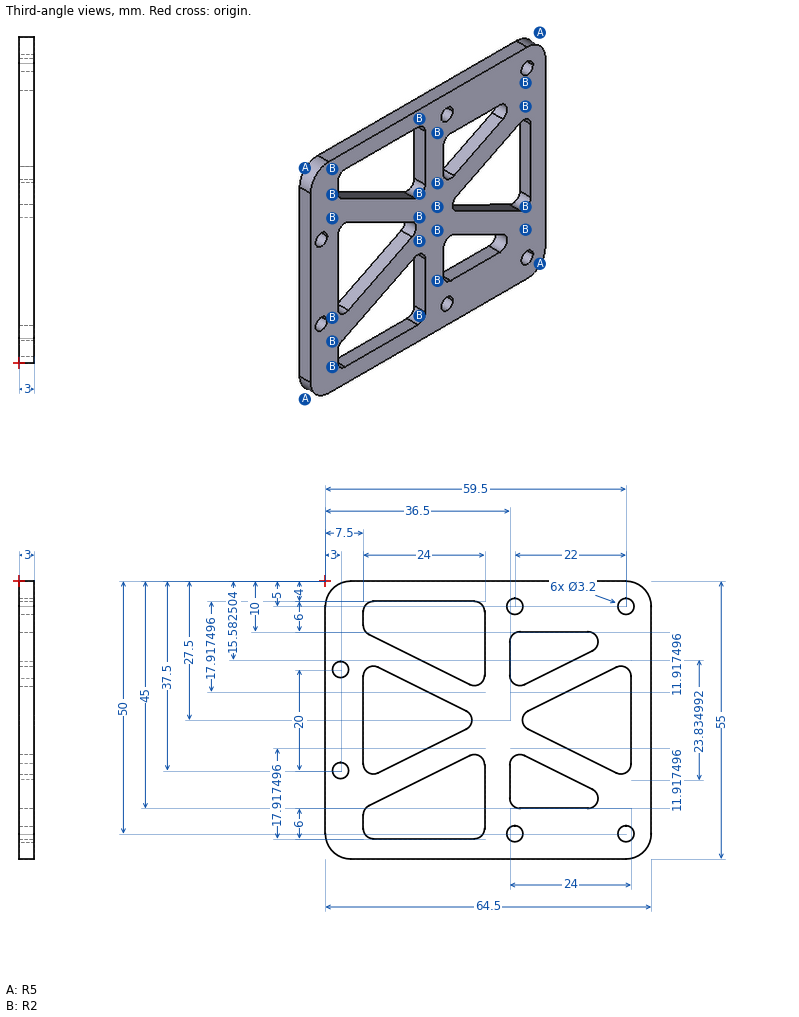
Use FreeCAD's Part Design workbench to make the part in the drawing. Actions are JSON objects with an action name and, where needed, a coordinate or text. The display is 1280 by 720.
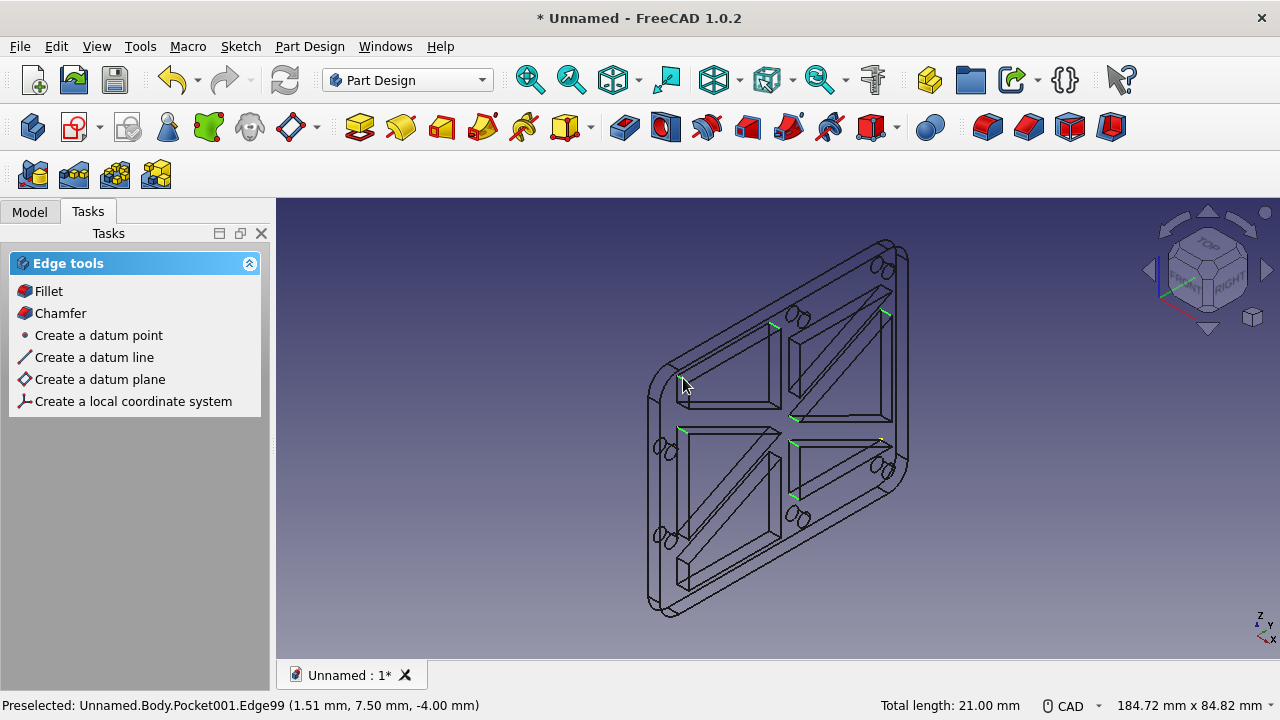
{"action": "left_click", "coordinate": [682, 404], "text": "ctrl"}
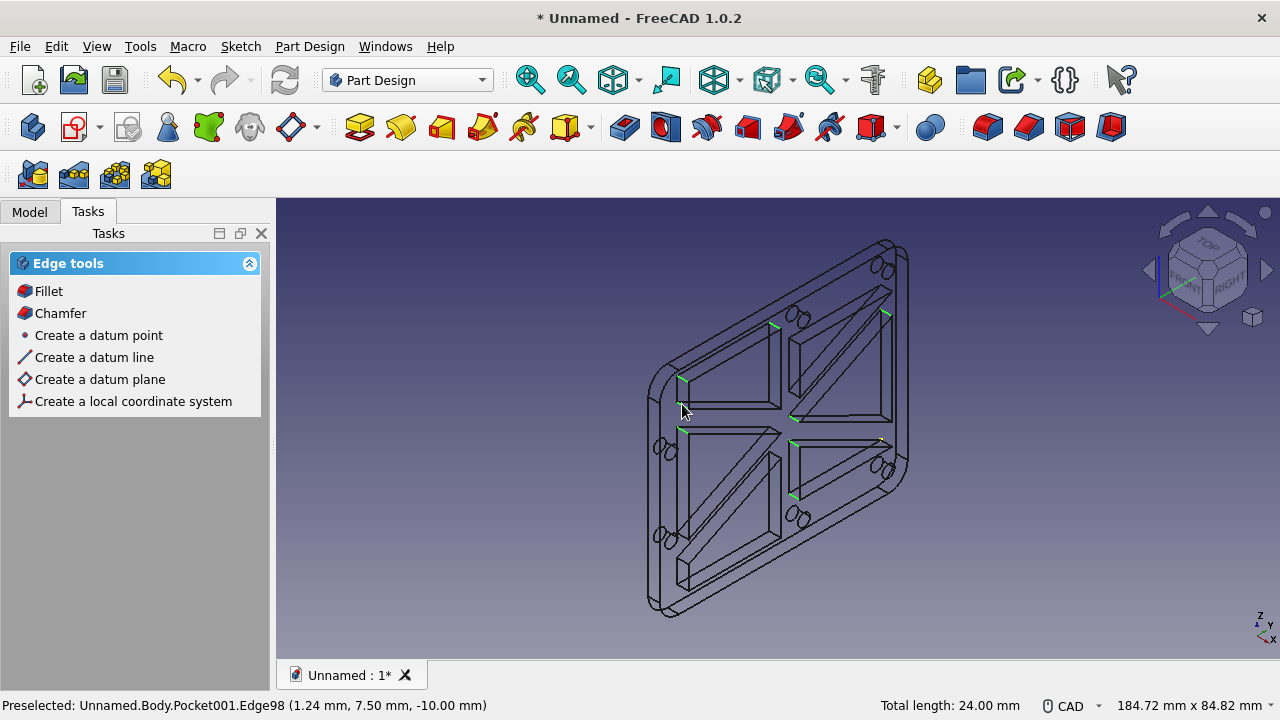
{"action": "left_click", "coordinate": [682, 586], "text": "ctrl"}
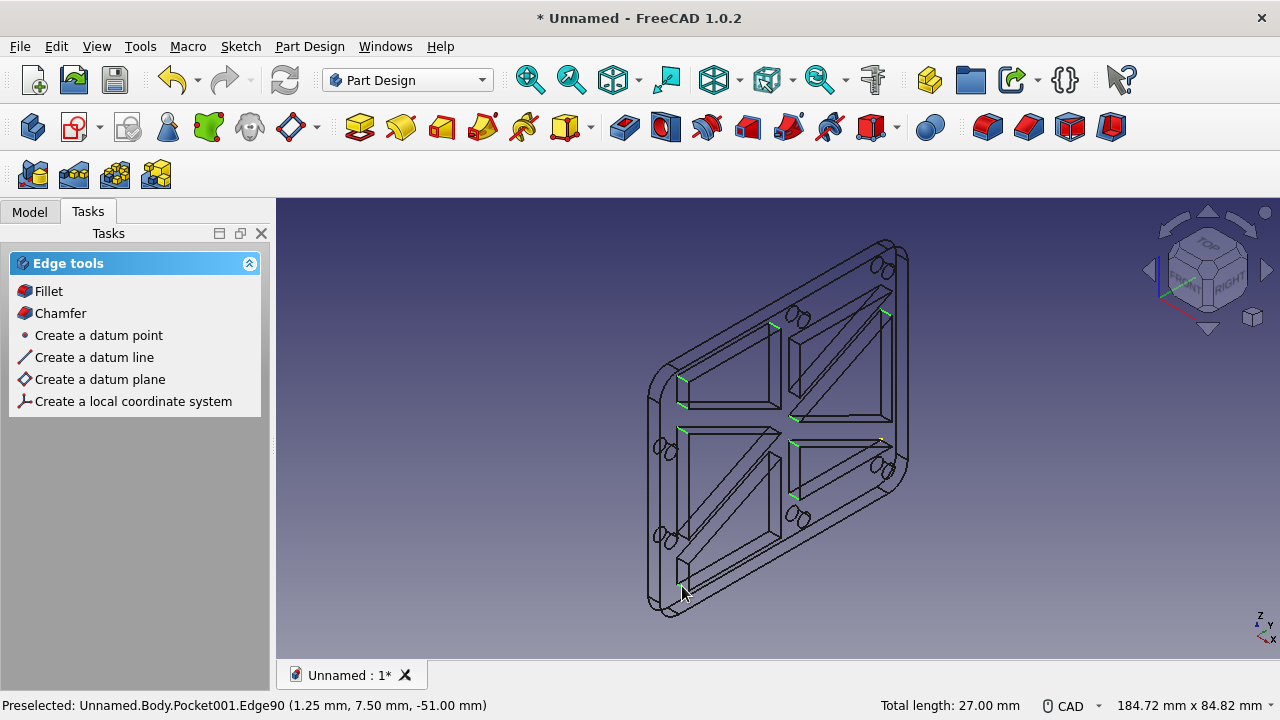
{"action": "left_click", "coordinate": [774, 533], "text": "ctrl"}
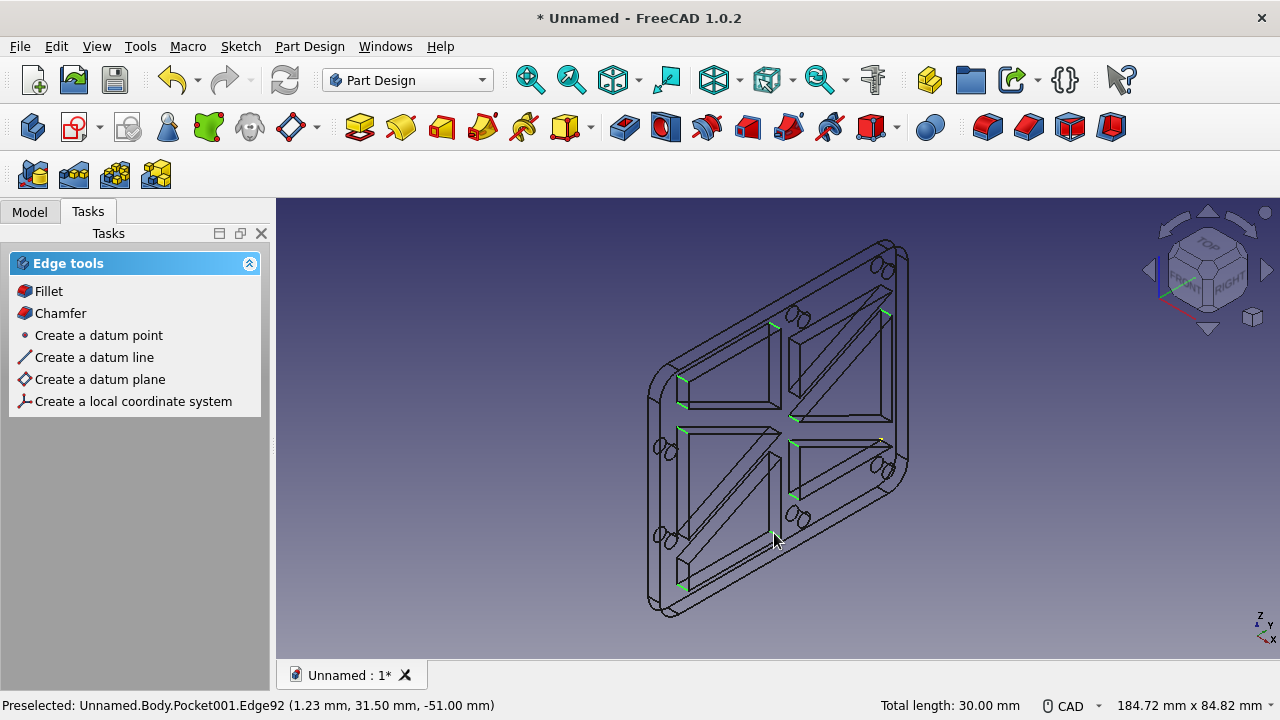
{"action": "left_click", "coordinate": [775, 454], "text": "ctrl"}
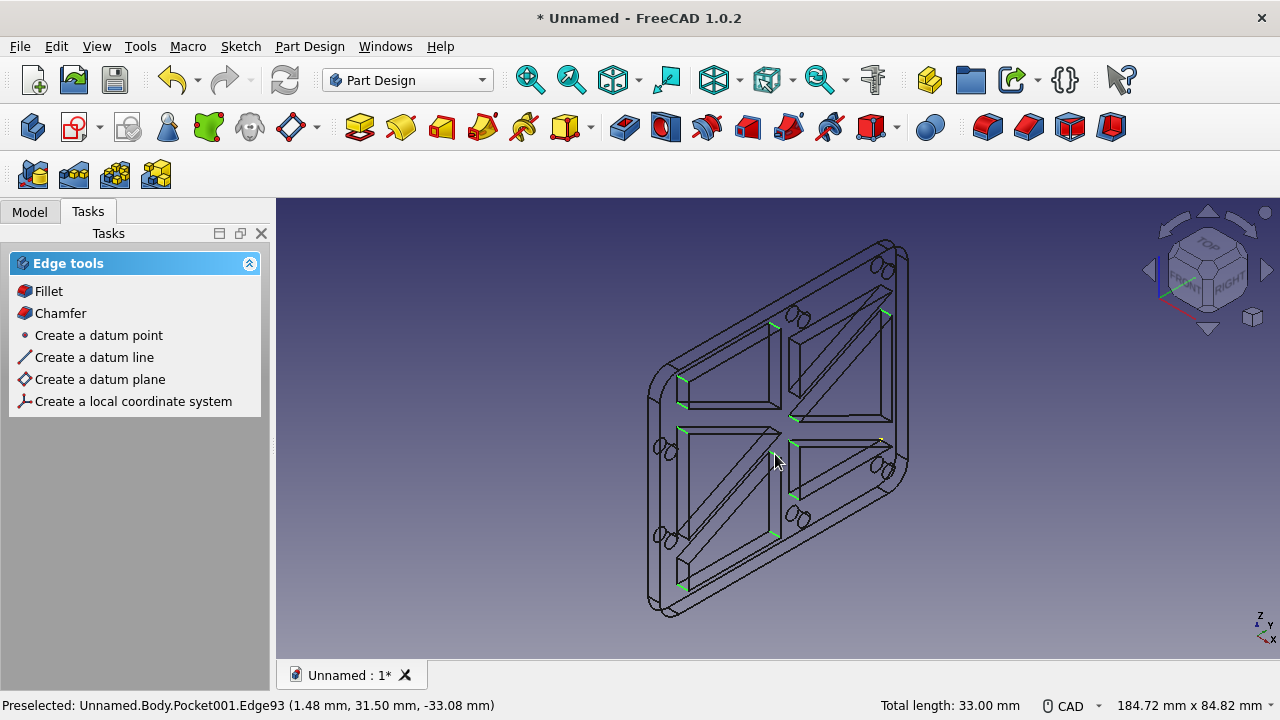
{"action": "left_click", "coordinate": [683, 560], "text": "ctrl"}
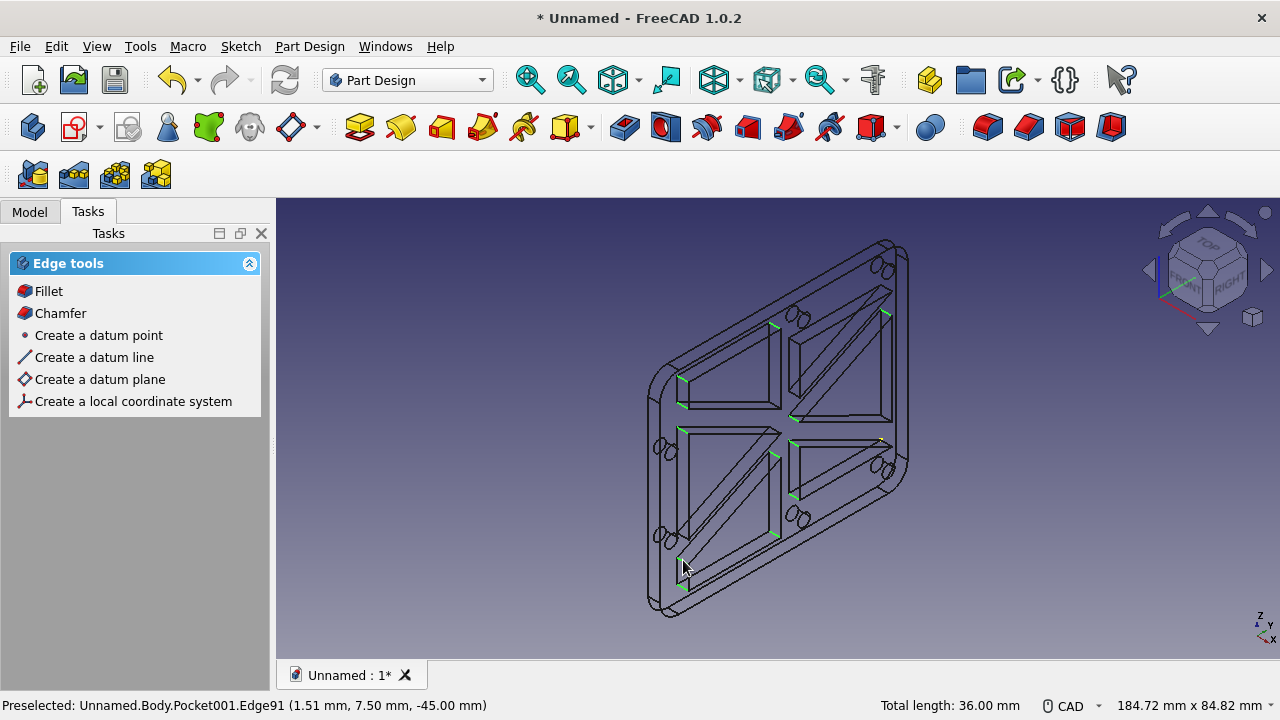
{"action": "left_click", "coordinate": [794, 340], "text": "ctrl"}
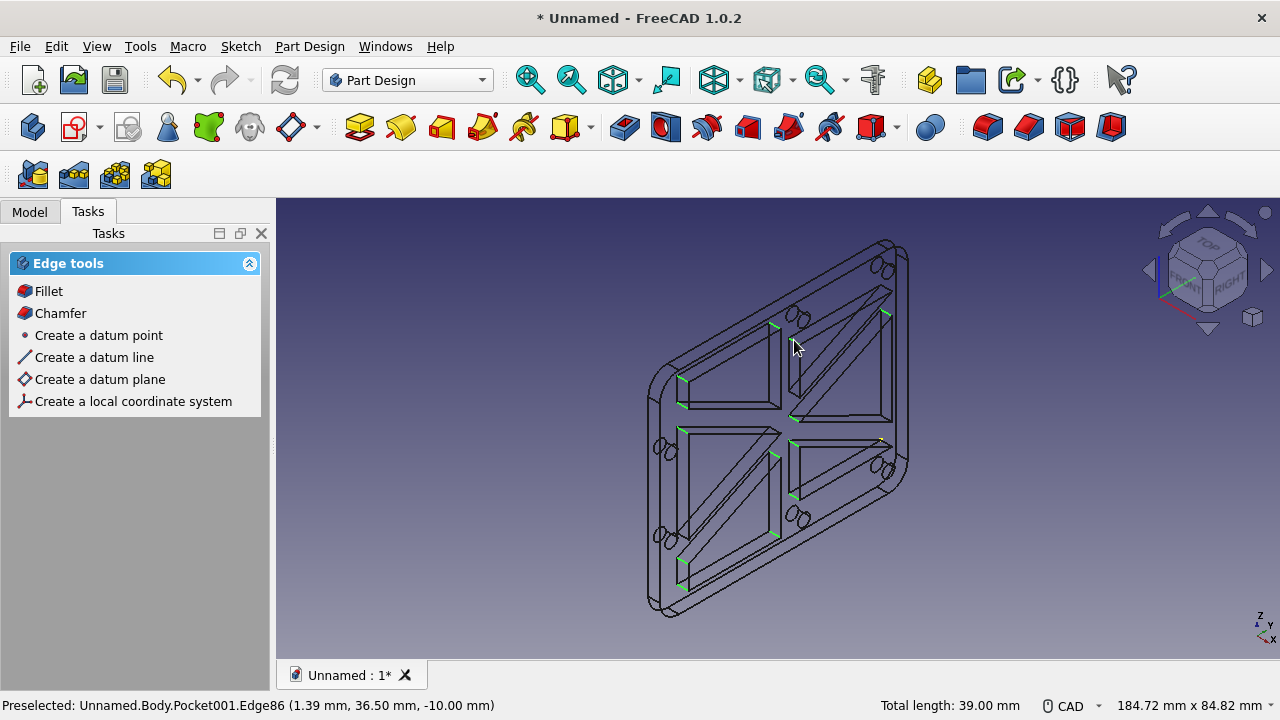
{"action": "left_click", "coordinate": [794, 393], "text": "ctrl"}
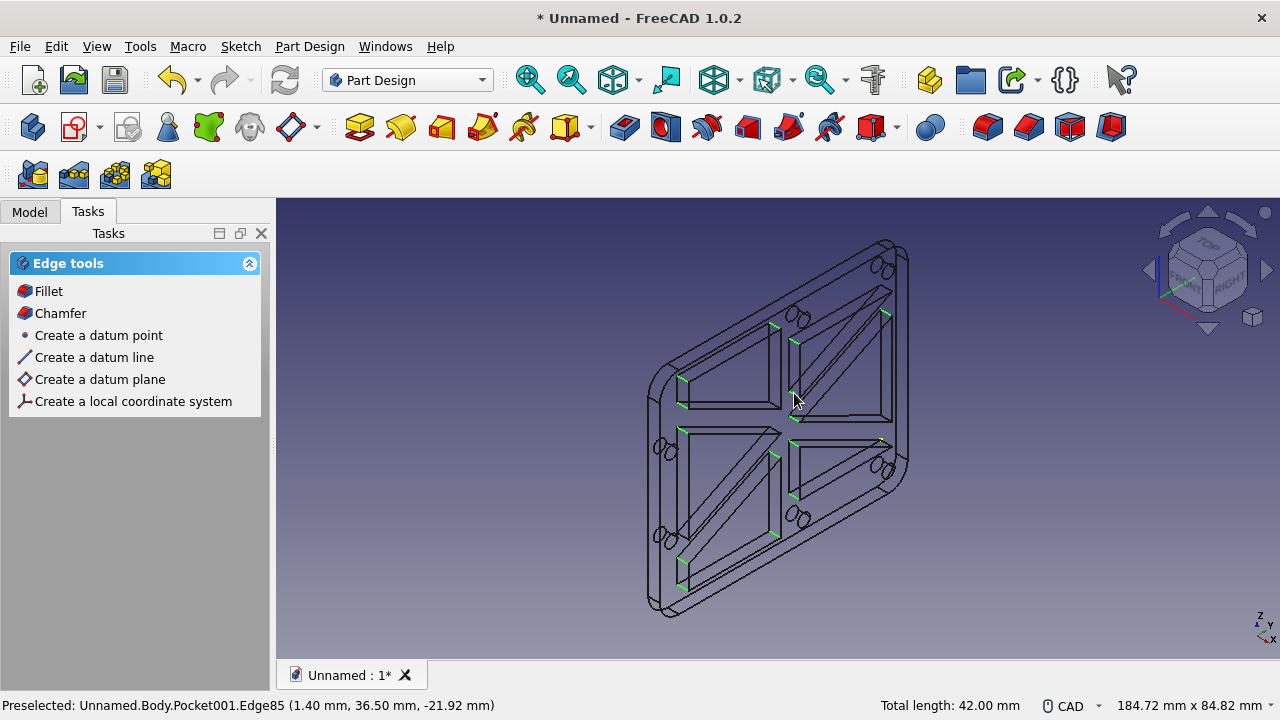
{"action": "left_click", "coordinate": [885, 286], "text": "ctrl"}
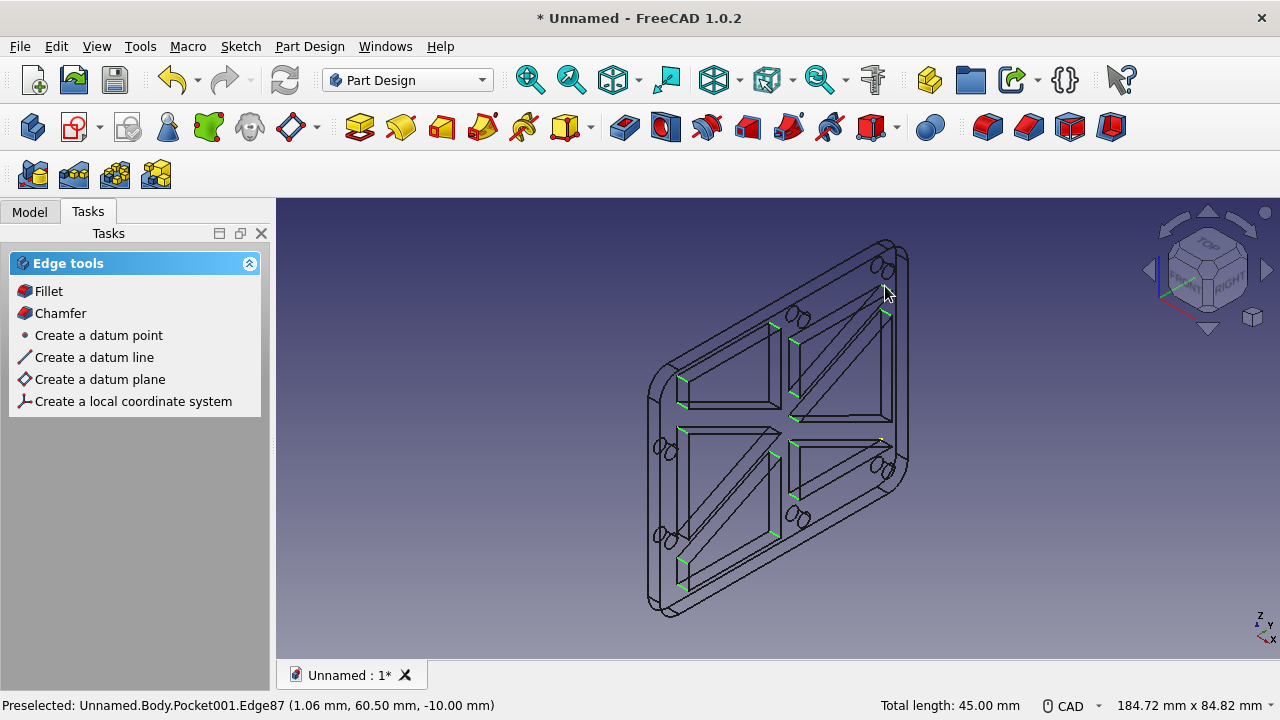
{"action": "scroll", "coordinate": [887, 442], "scroll_direction": "up", "scroll_amount": 5}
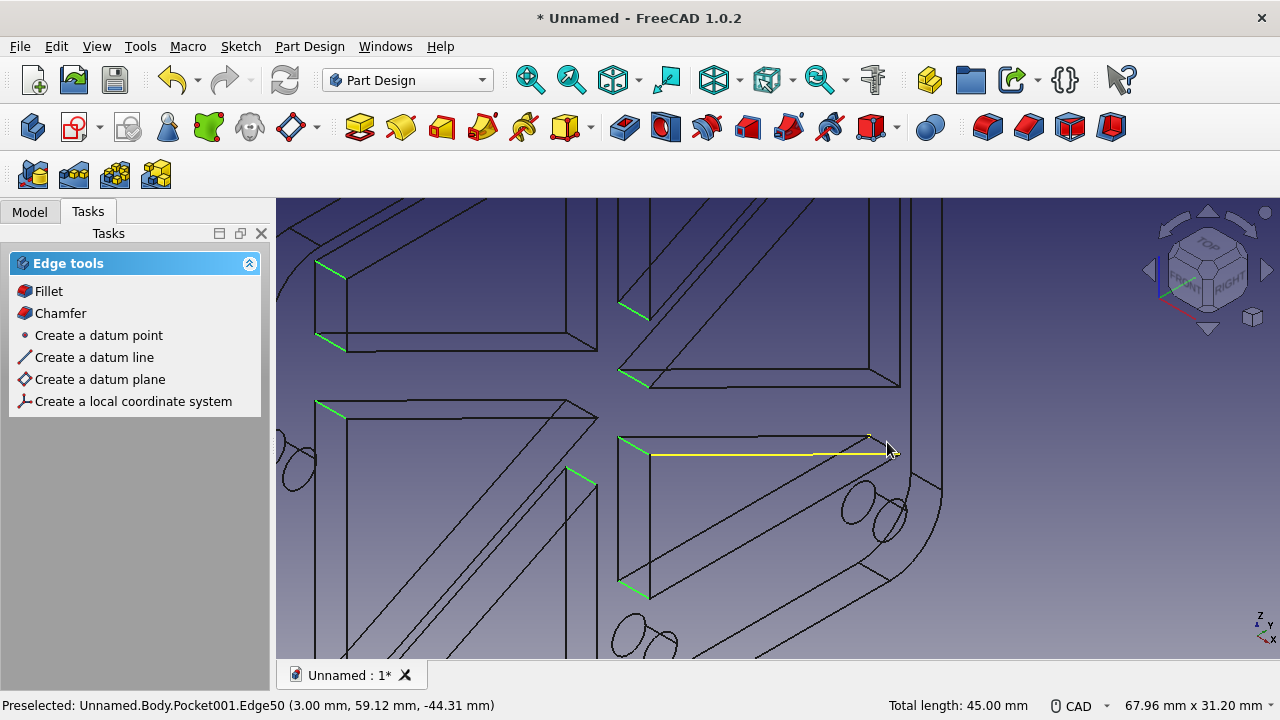
{"action": "left_click", "coordinate": [885, 444], "text": "ctrl"}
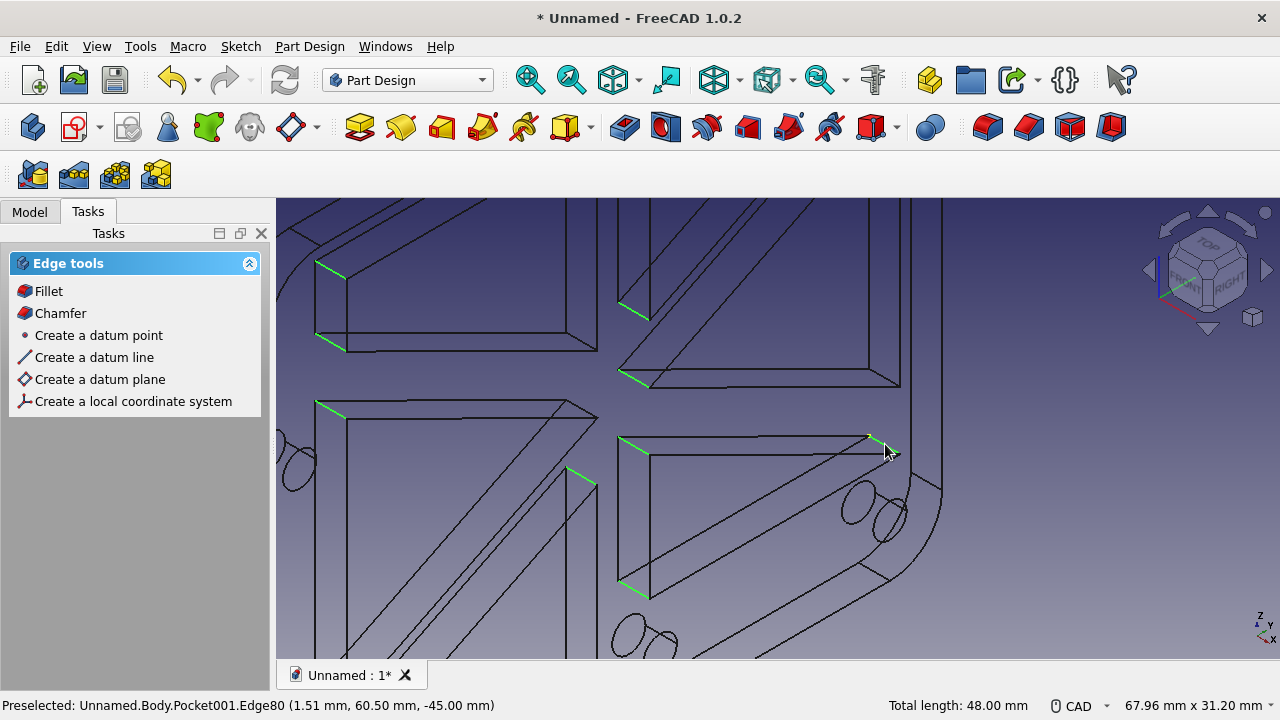
{"action": "left_click", "coordinate": [885, 377], "text": "ctrl"}